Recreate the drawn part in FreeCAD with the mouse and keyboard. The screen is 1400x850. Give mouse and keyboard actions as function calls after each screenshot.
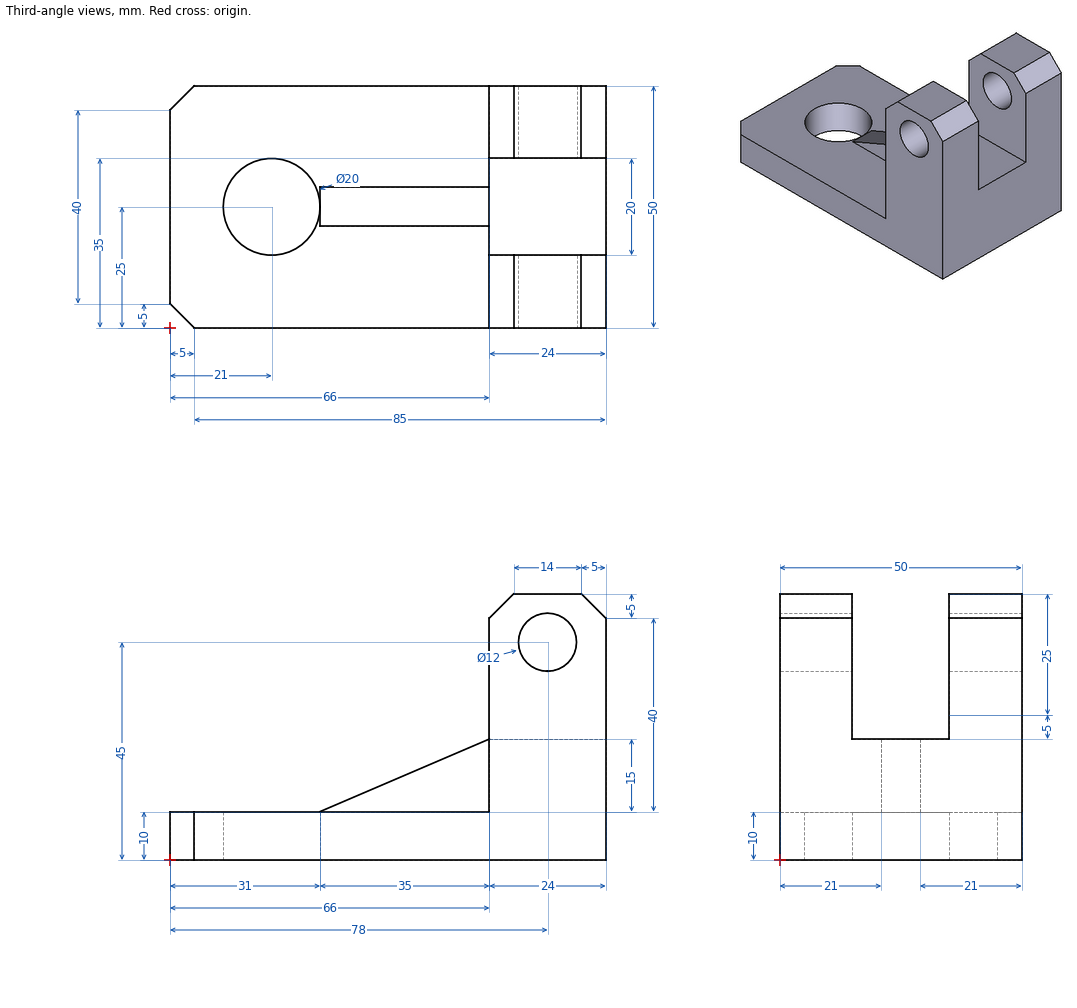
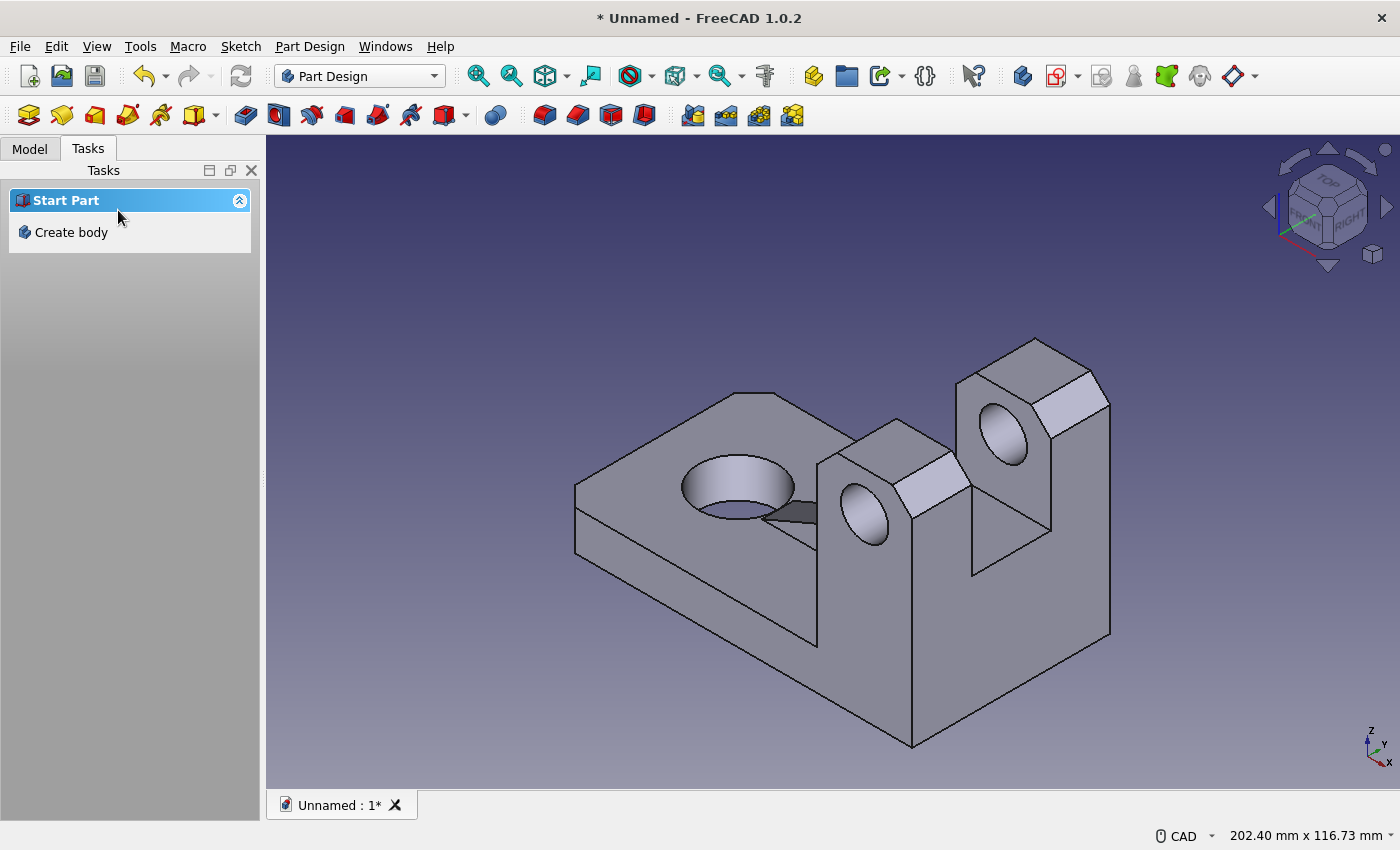
click(989, 526)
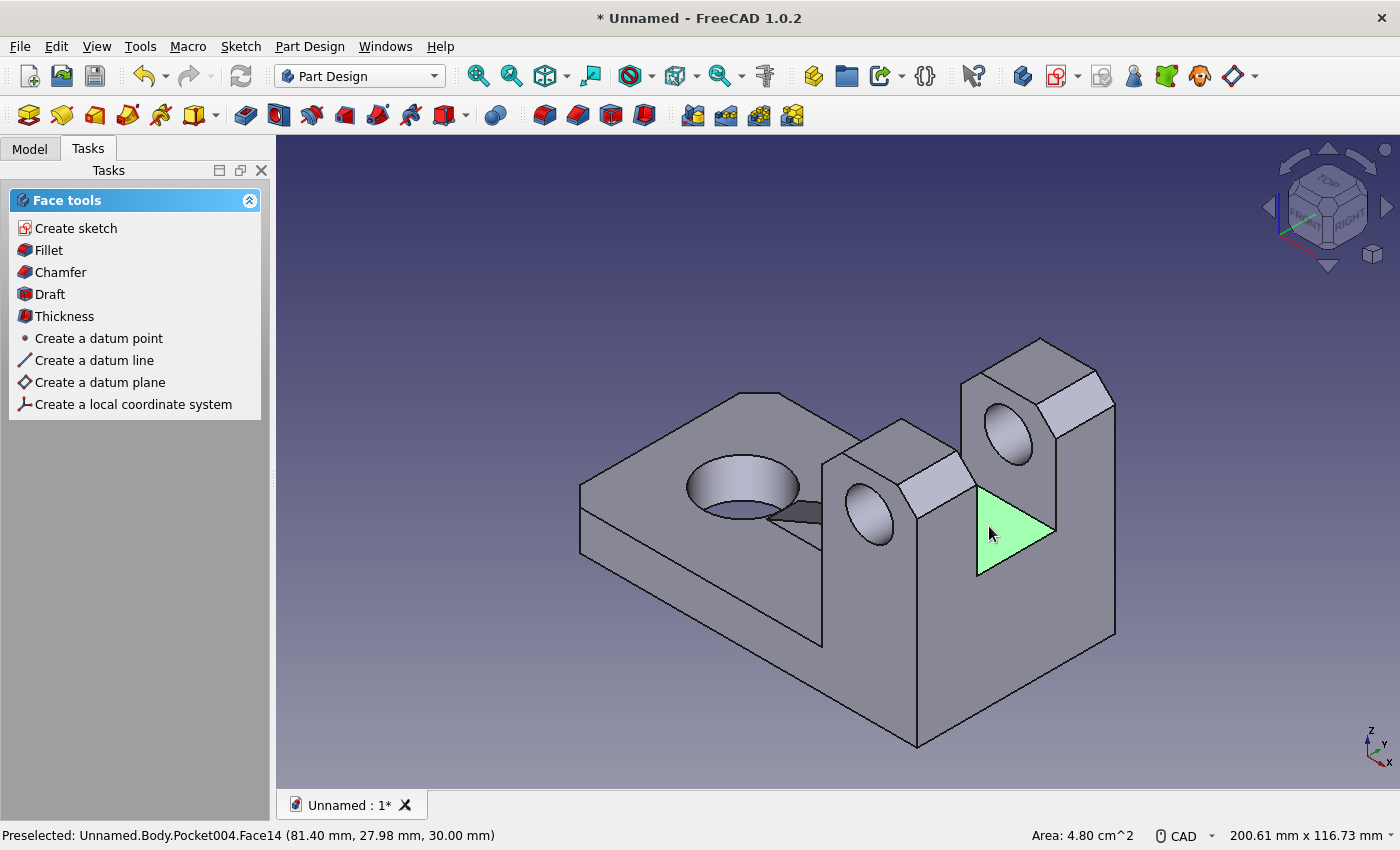
click(1056, 76)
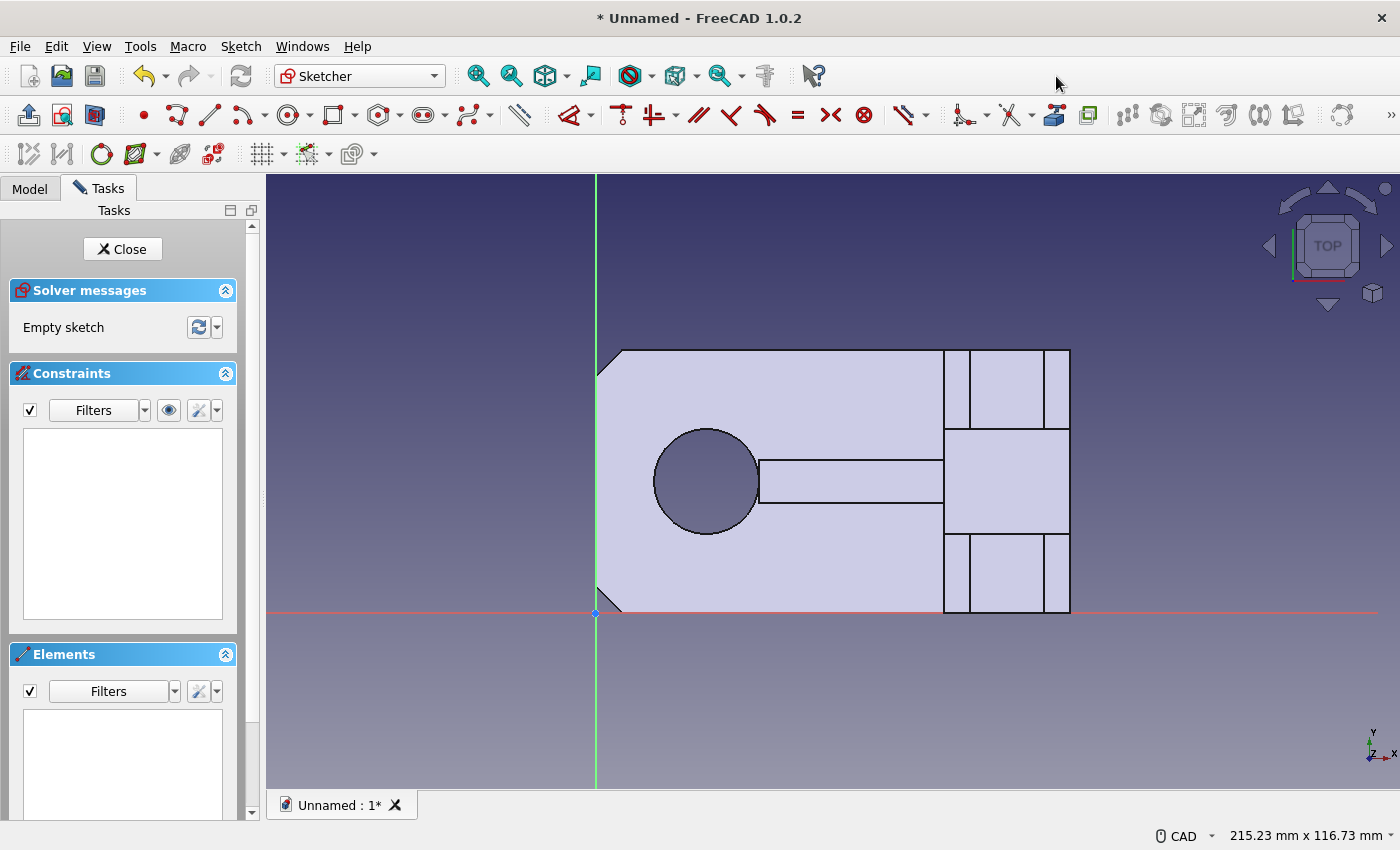
click(95, 116)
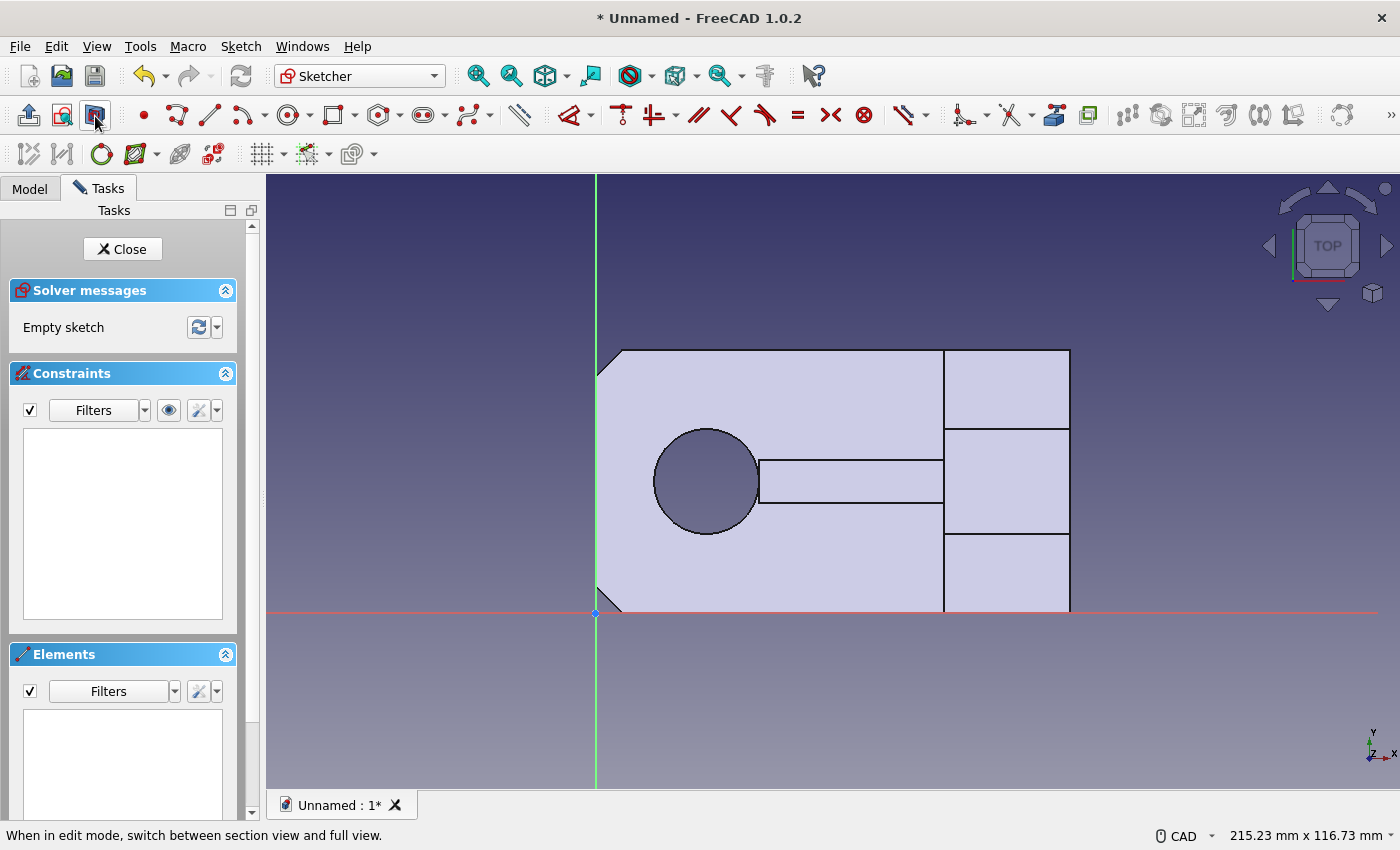
scroll(1086, 481, up, 7)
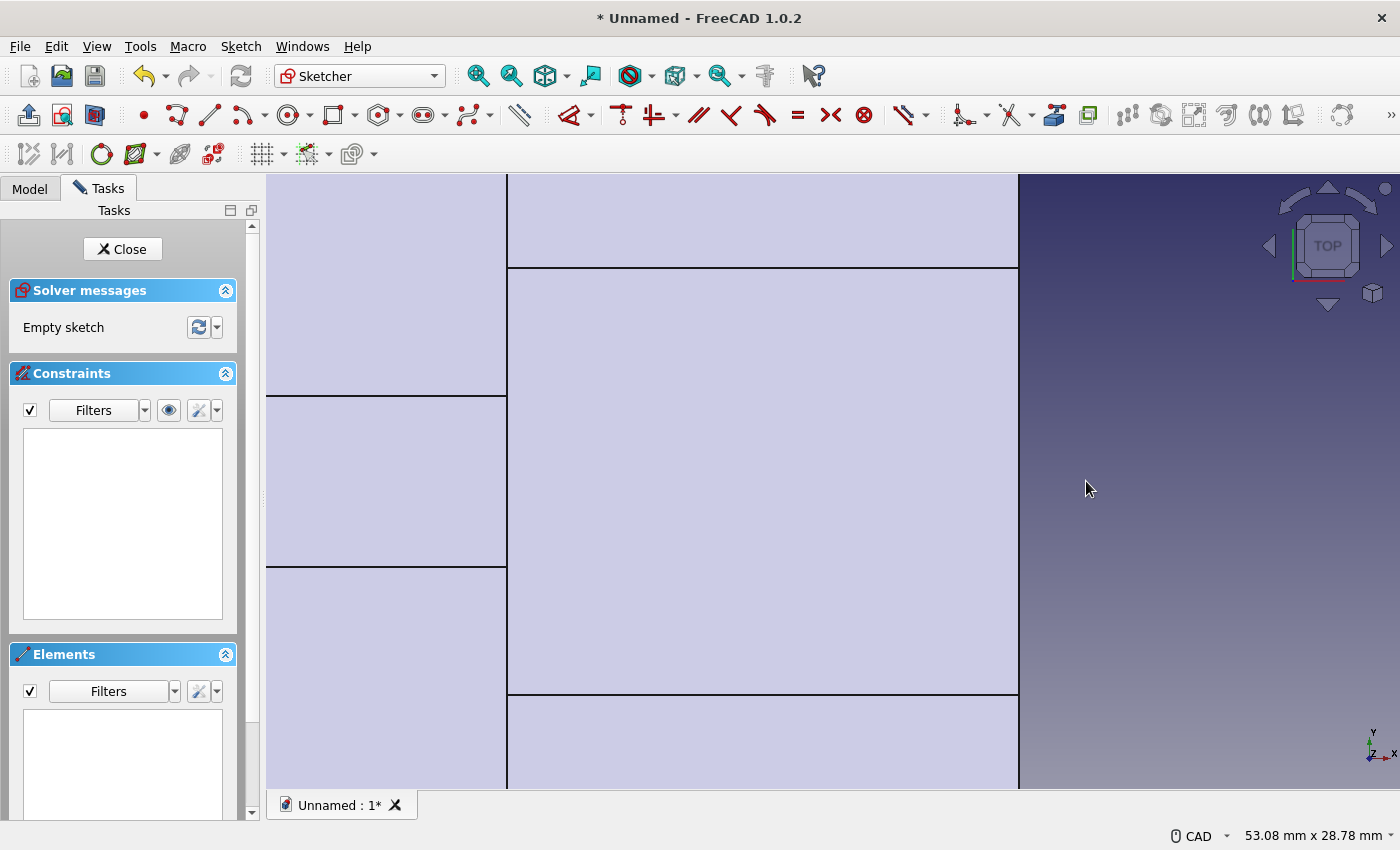
click(332, 116)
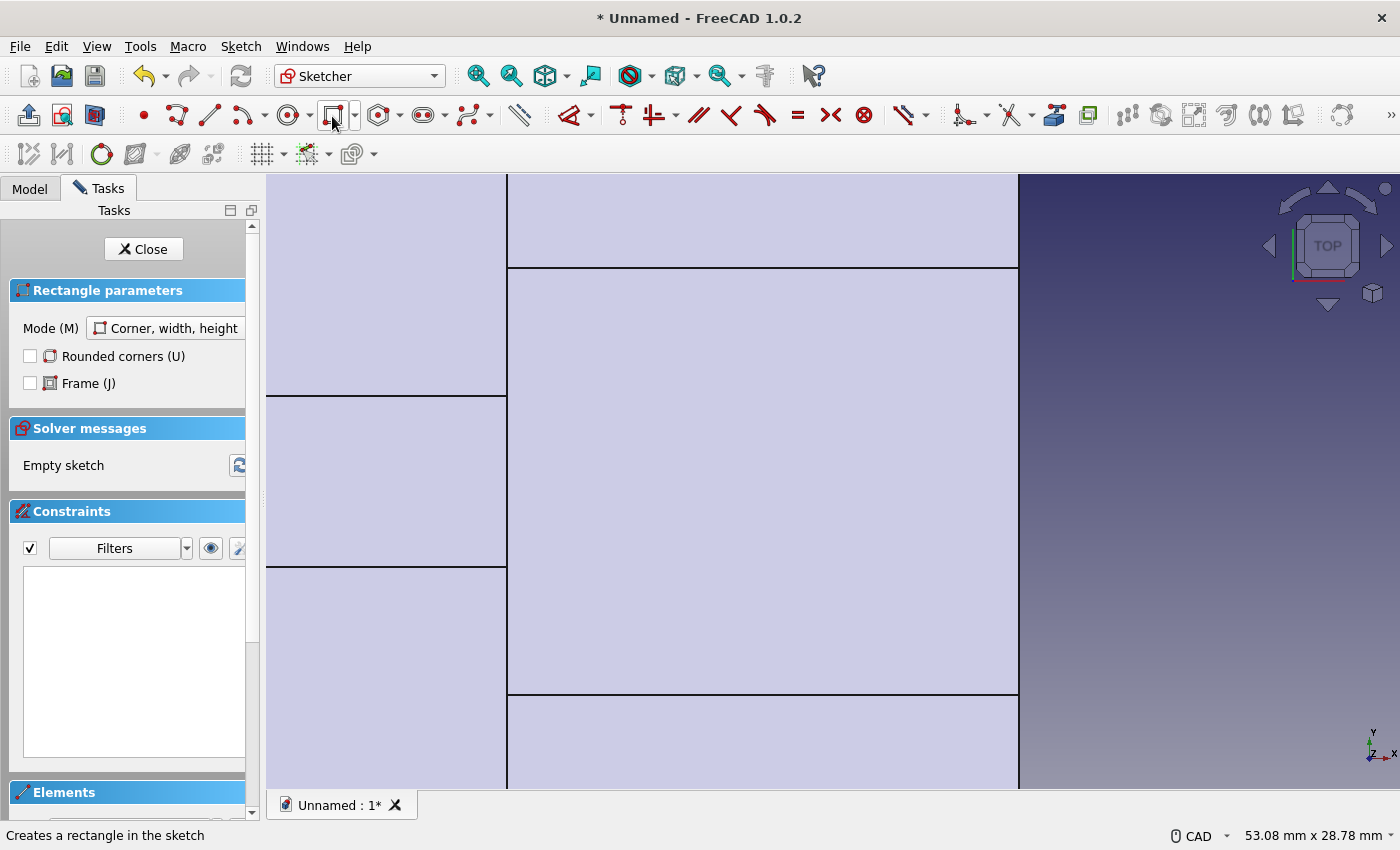
click(507, 268)
move(1019, 695)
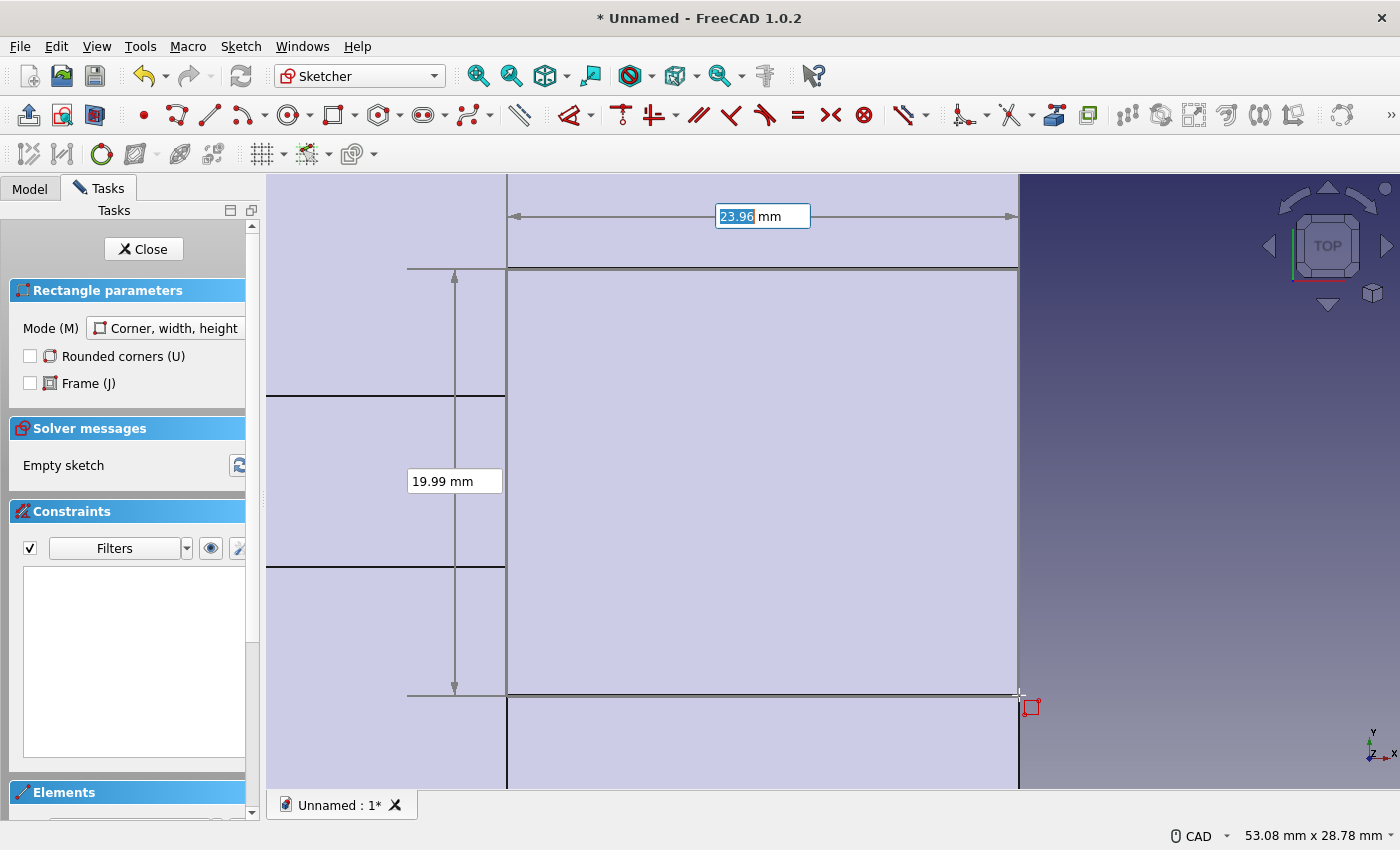
text(24)
key(Tab)
text(20)
key(Return)
key(Escape)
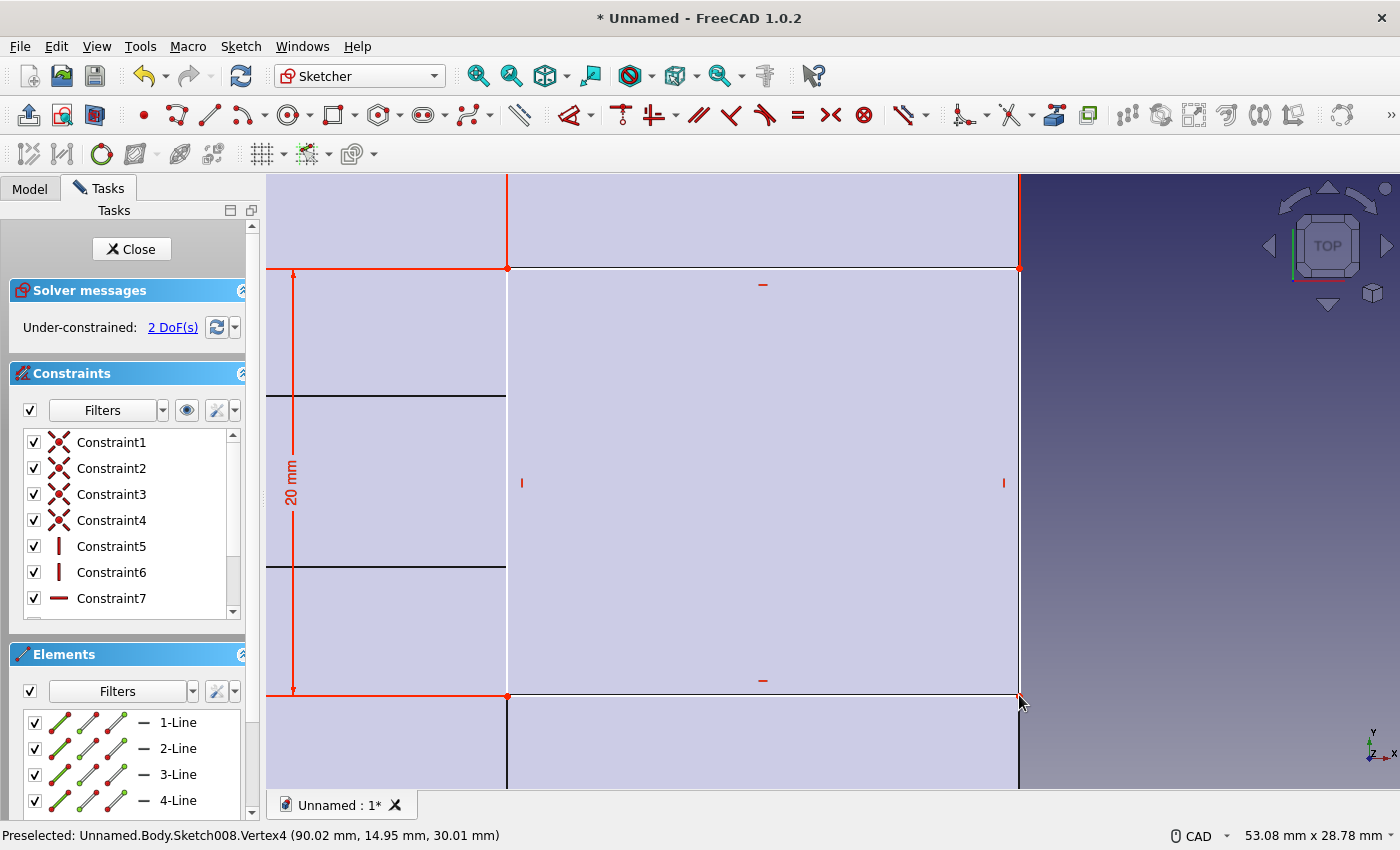
click(568, 116)